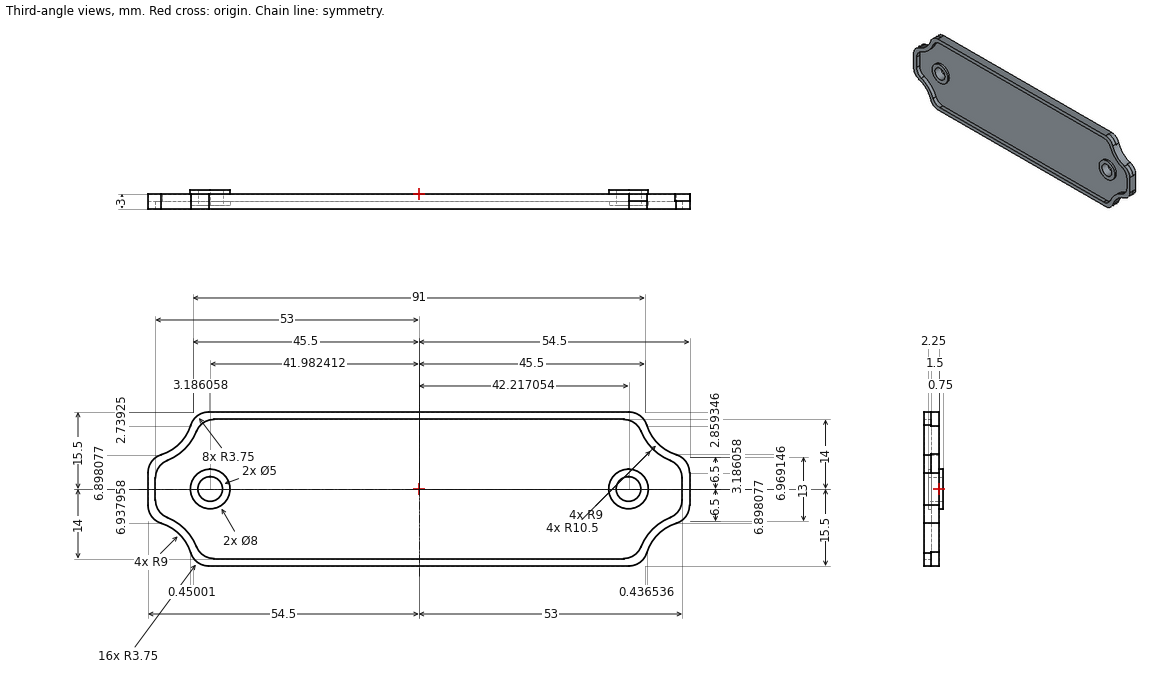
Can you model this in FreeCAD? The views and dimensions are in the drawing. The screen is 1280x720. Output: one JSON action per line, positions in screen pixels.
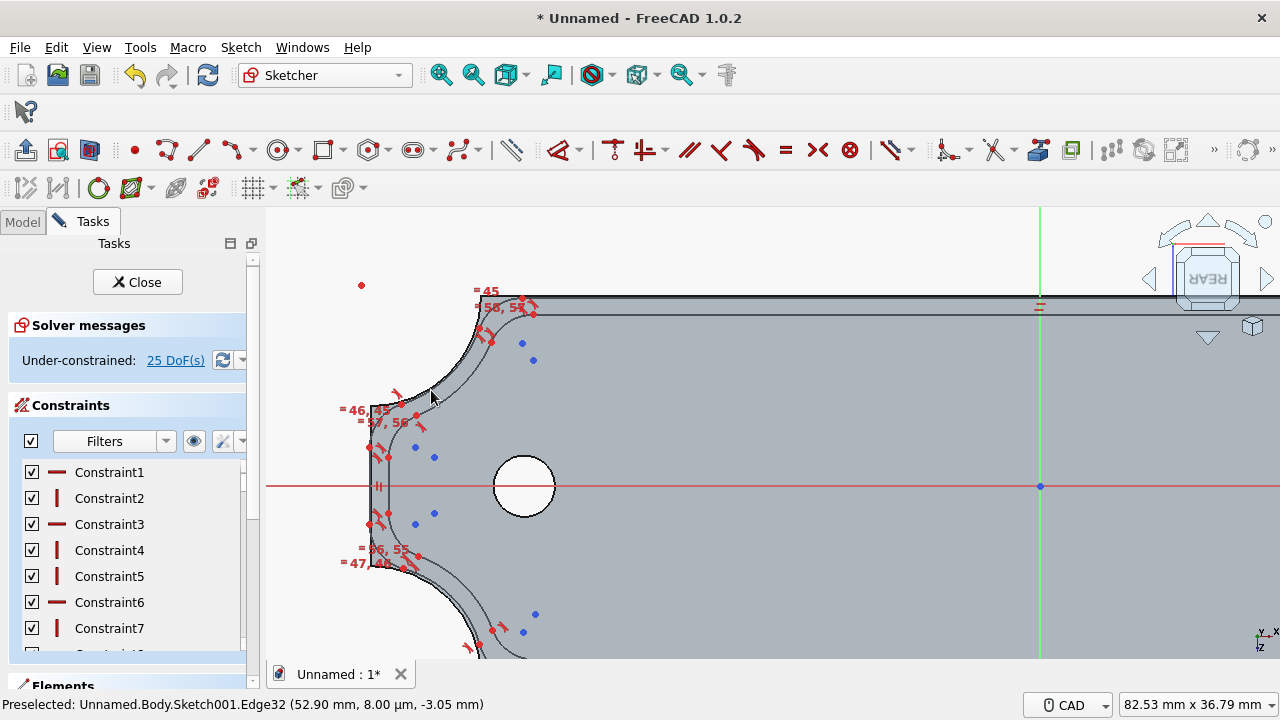
{"action": "left_click", "coordinate": [432, 390]}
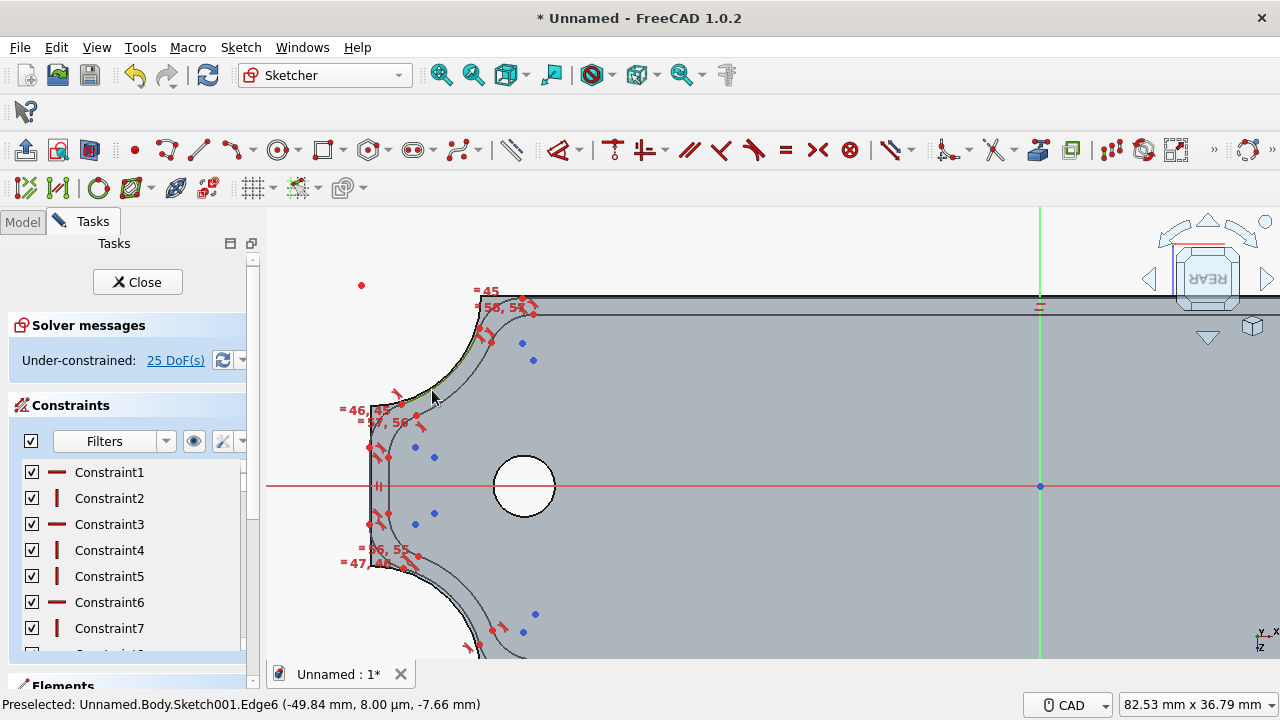
{"action": "left_click", "coordinate": [466, 614]}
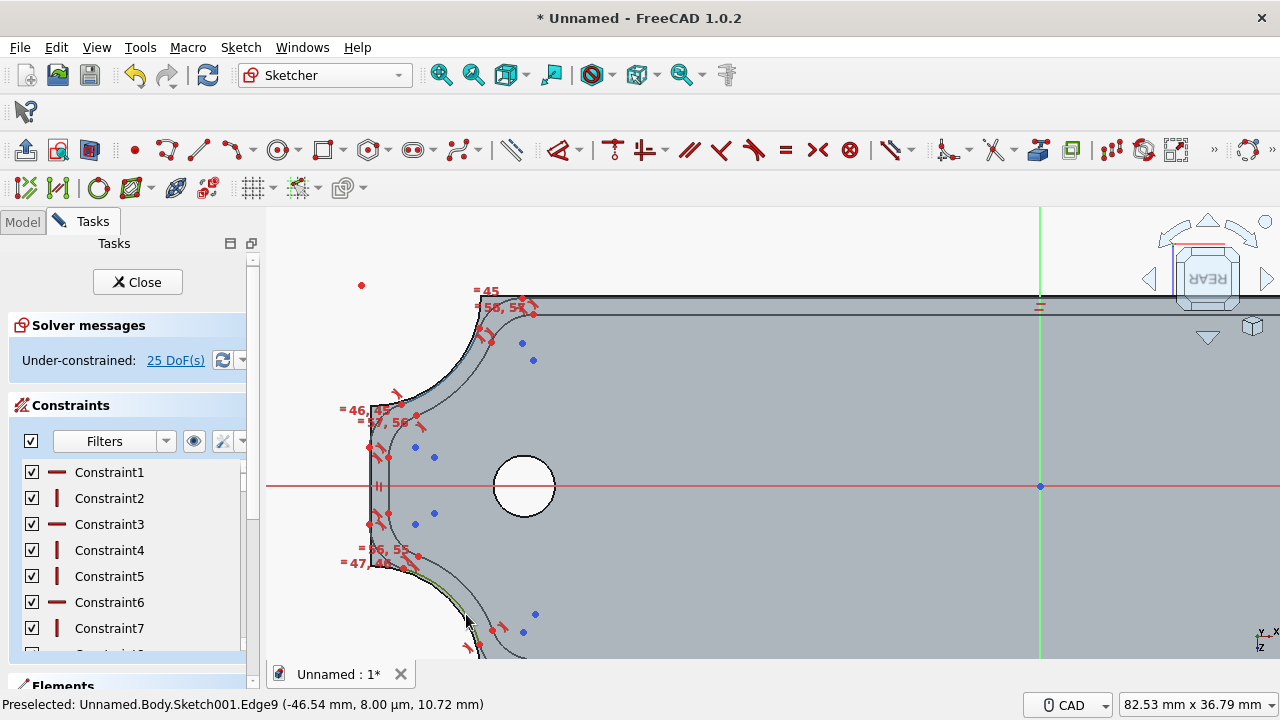
{"action": "scroll", "coordinate": [431, 390], "scroll_direction": "down", "scroll_amount": 4}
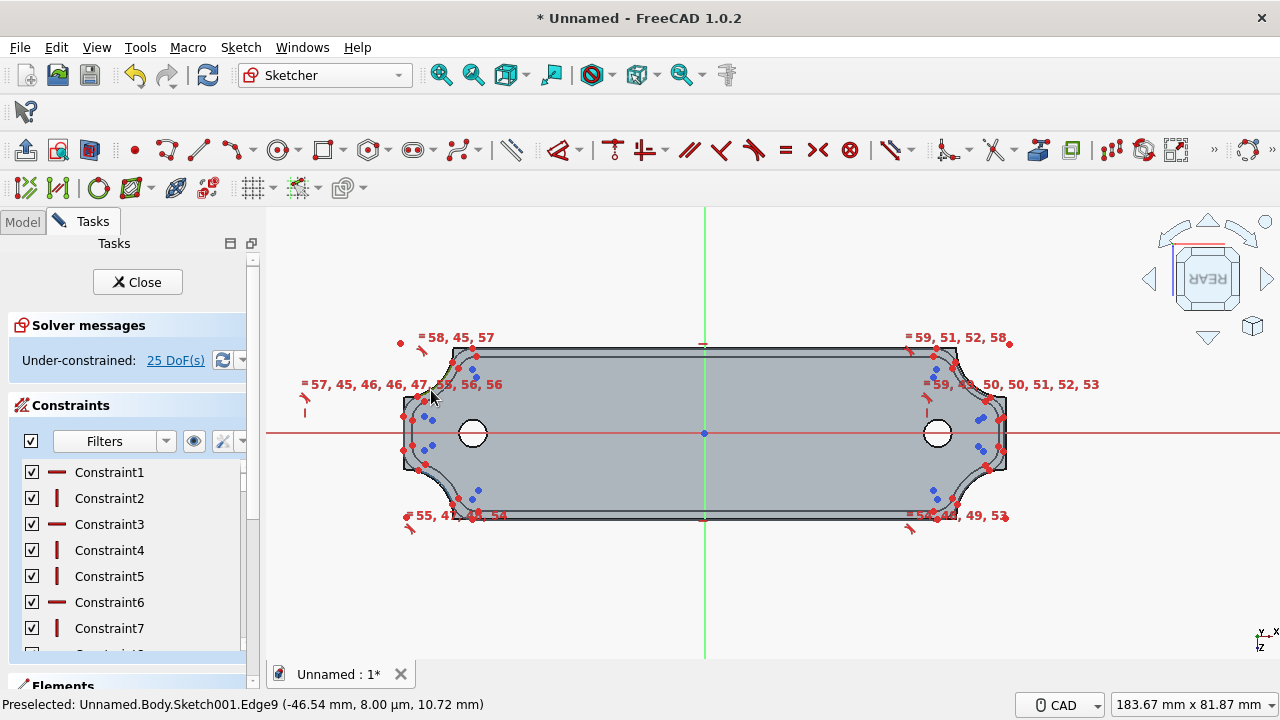
{"action": "scroll", "coordinate": [977, 477], "scroll_direction": "up", "scroll_amount": 4}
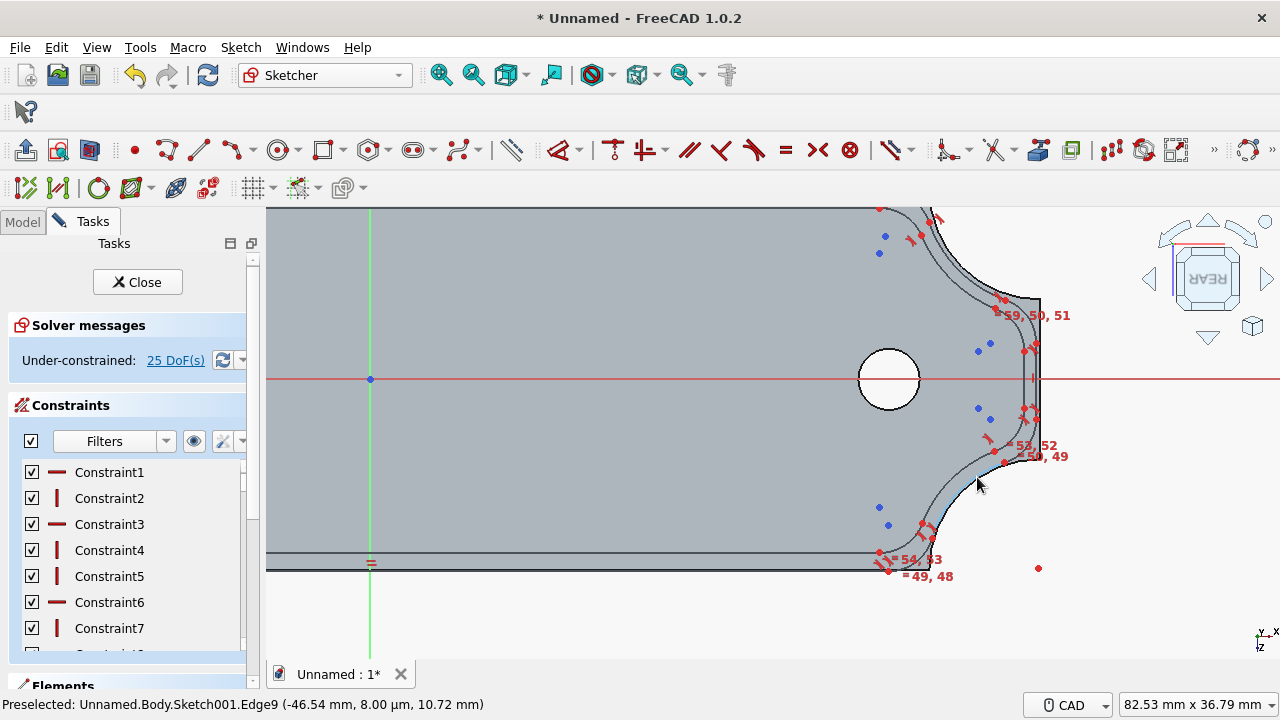
{"action": "left_click", "coordinate": [975, 477]}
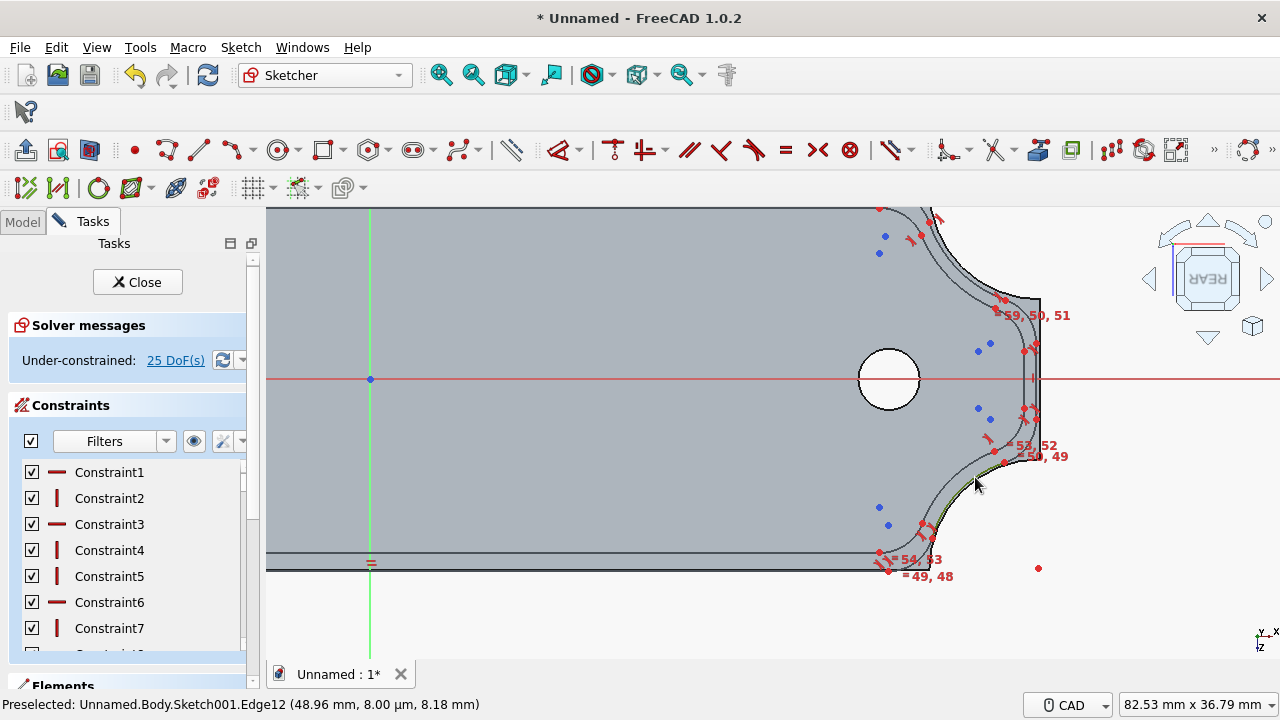
{"action": "left_click", "coordinate": [944, 253]}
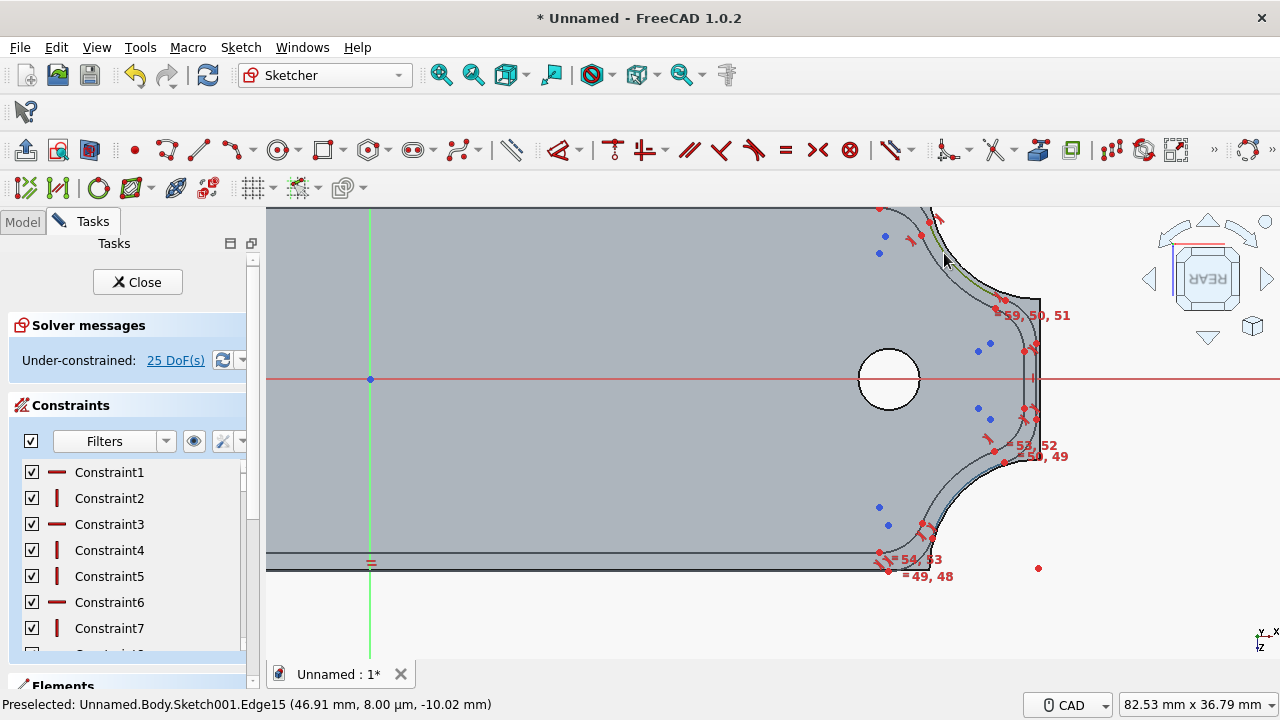
{"action": "left_click", "coordinate": [786, 150]}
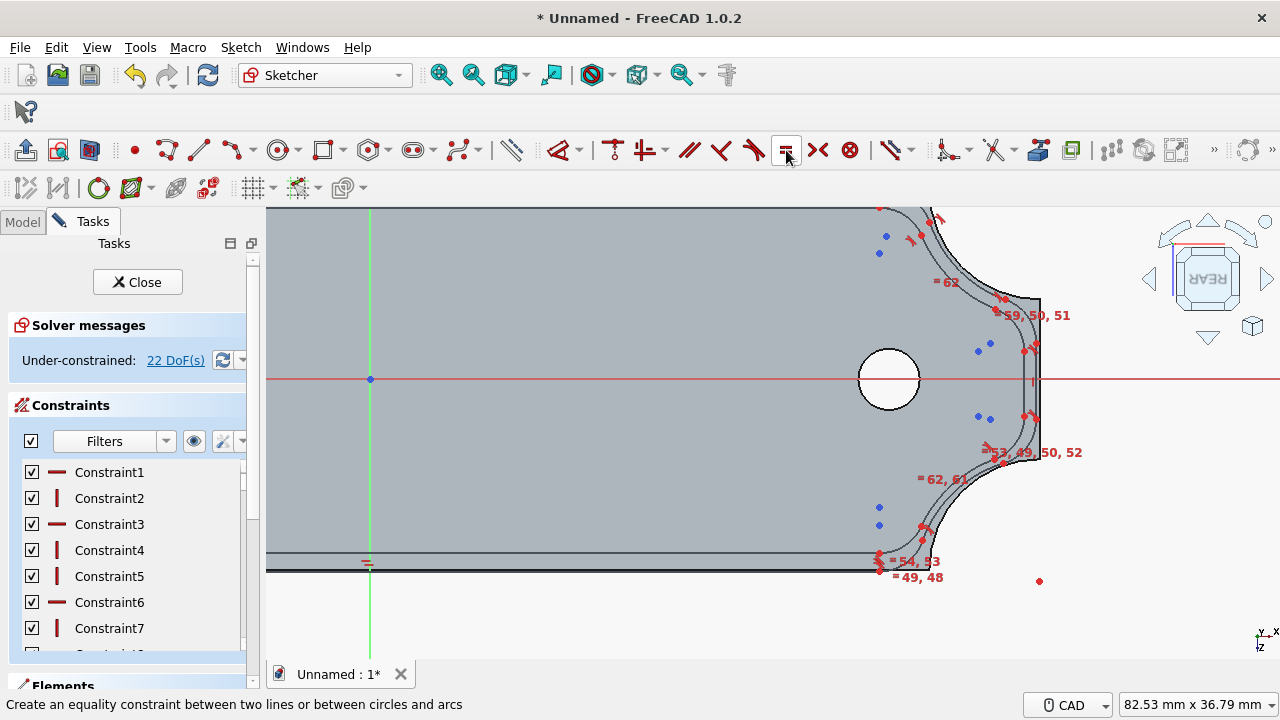
{"action": "scroll", "coordinate": [931, 509], "scroll_direction": "up", "scroll_amount": 4}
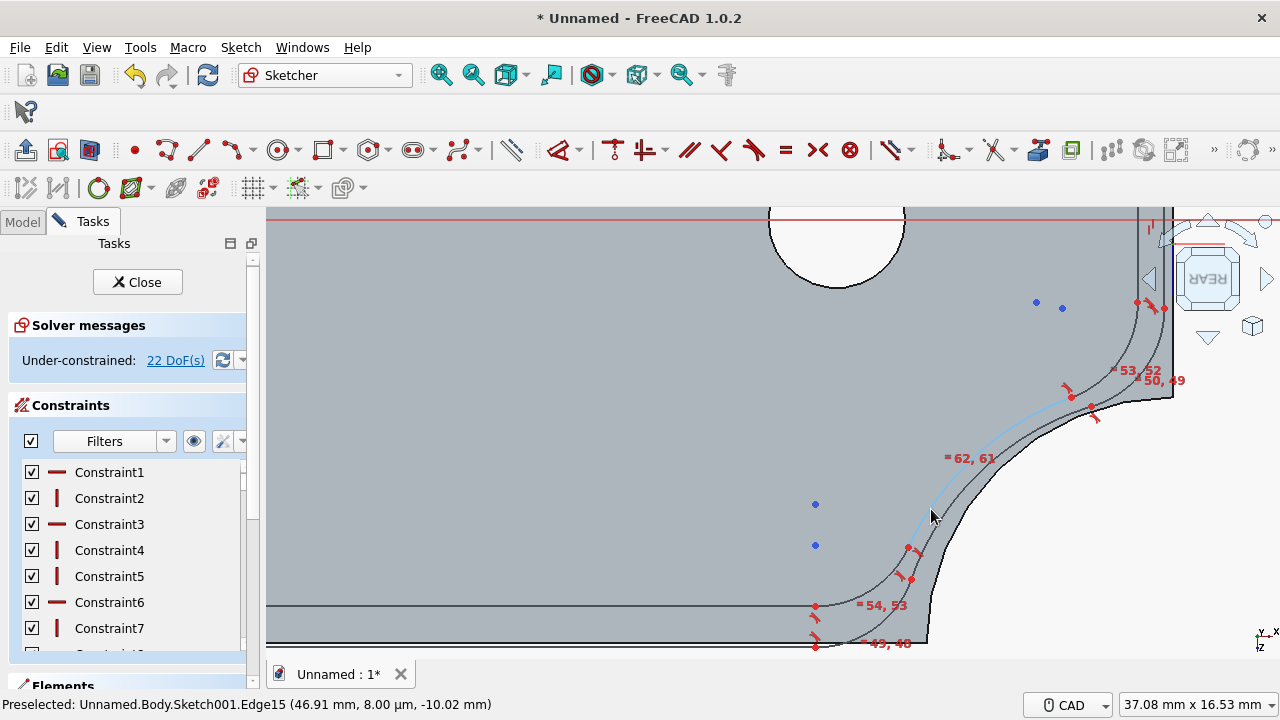
{"action": "left_click", "coordinate": [931, 508]}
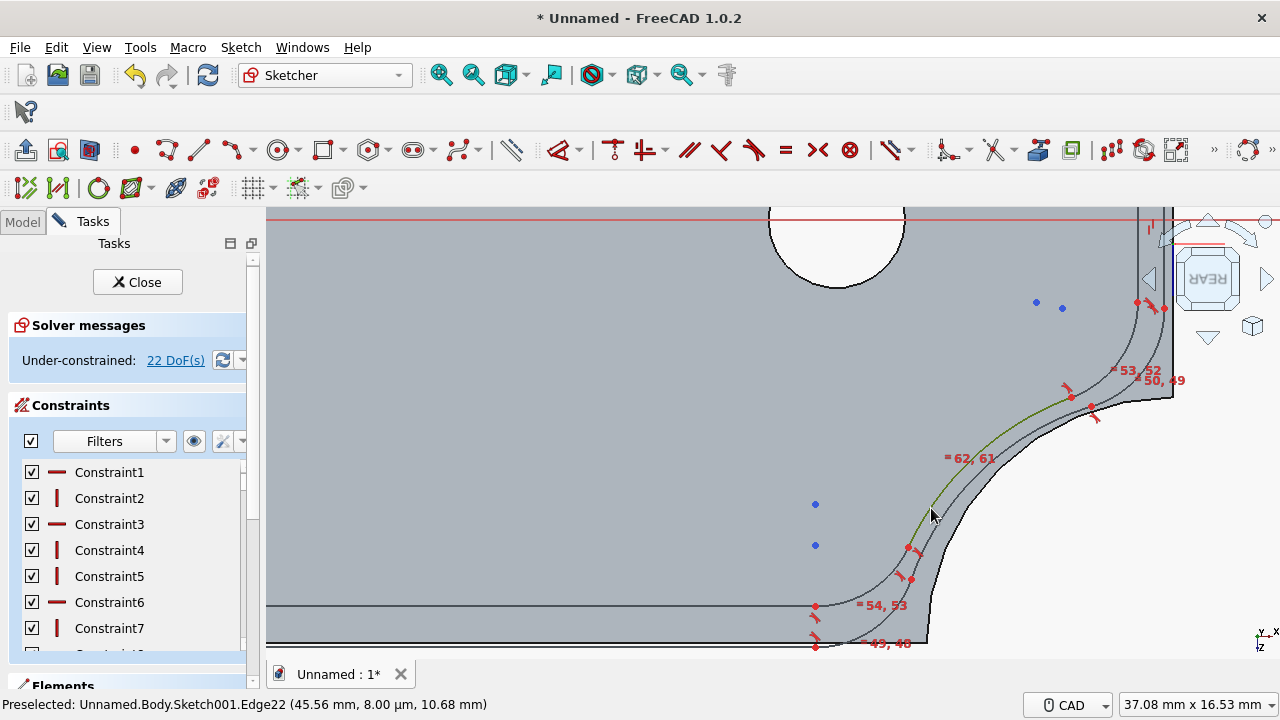
{"action": "scroll", "coordinate": [963, 487], "scroll_direction": "down", "scroll_amount": 8}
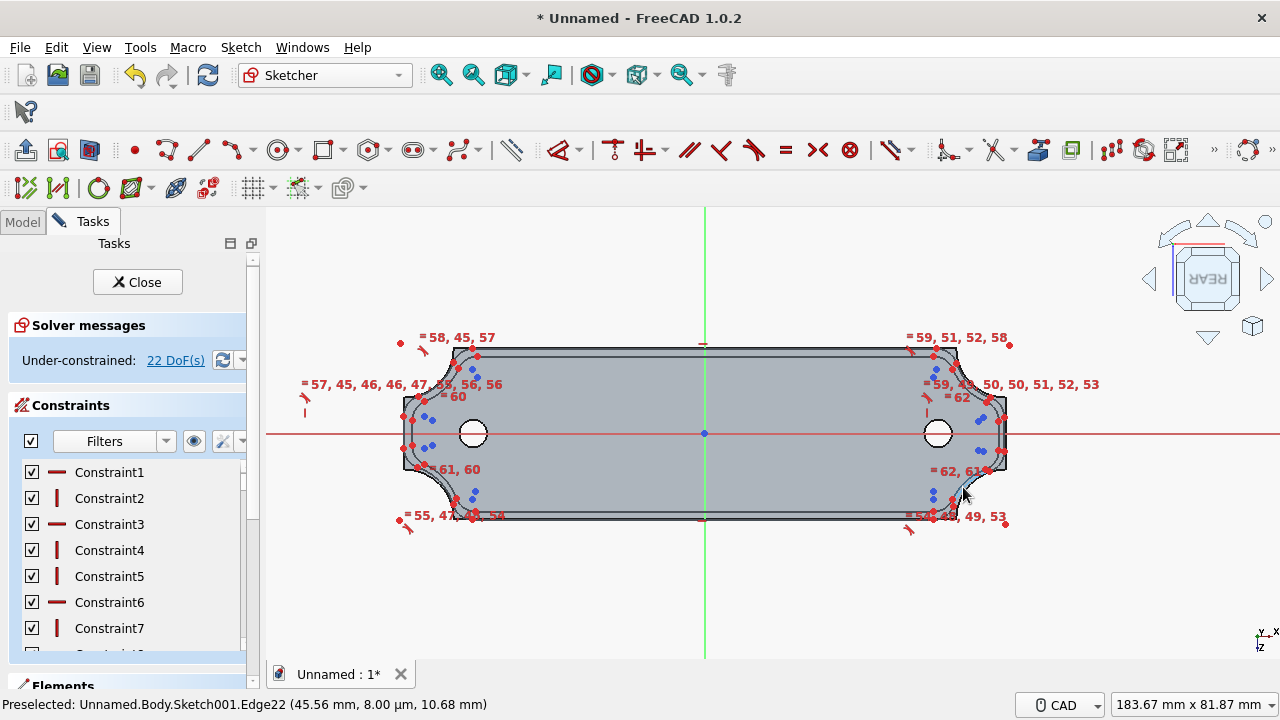
{"action": "scroll", "coordinate": [450, 486], "scroll_direction": "up", "scroll_amount": 5}